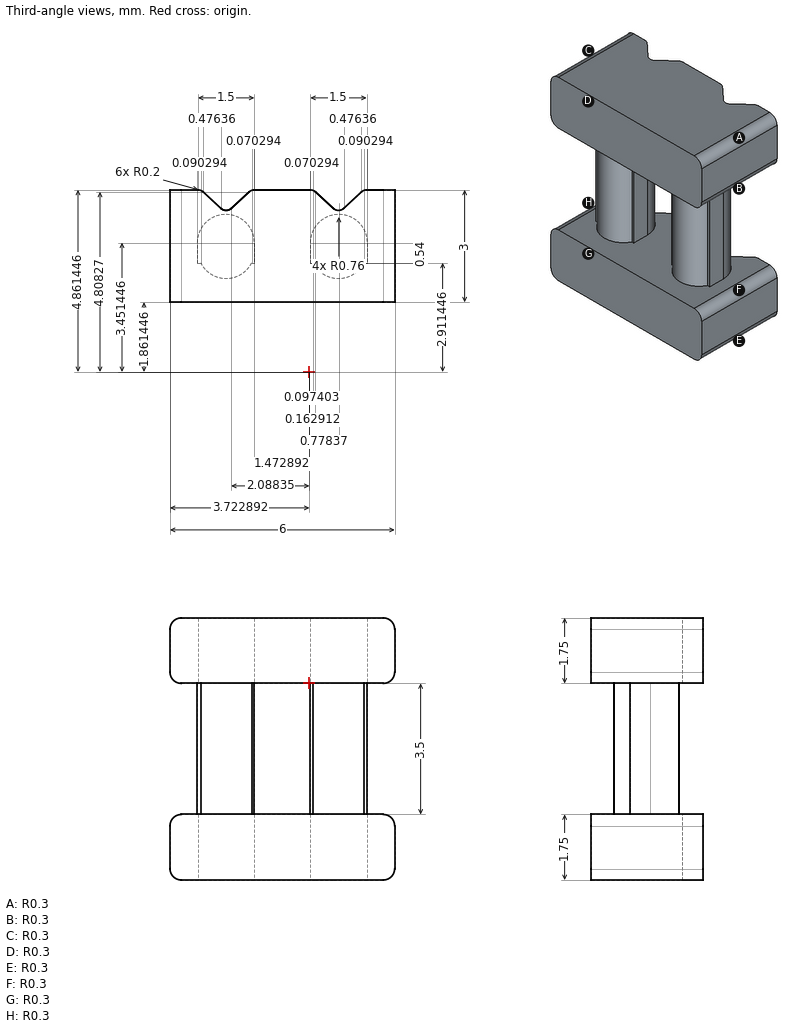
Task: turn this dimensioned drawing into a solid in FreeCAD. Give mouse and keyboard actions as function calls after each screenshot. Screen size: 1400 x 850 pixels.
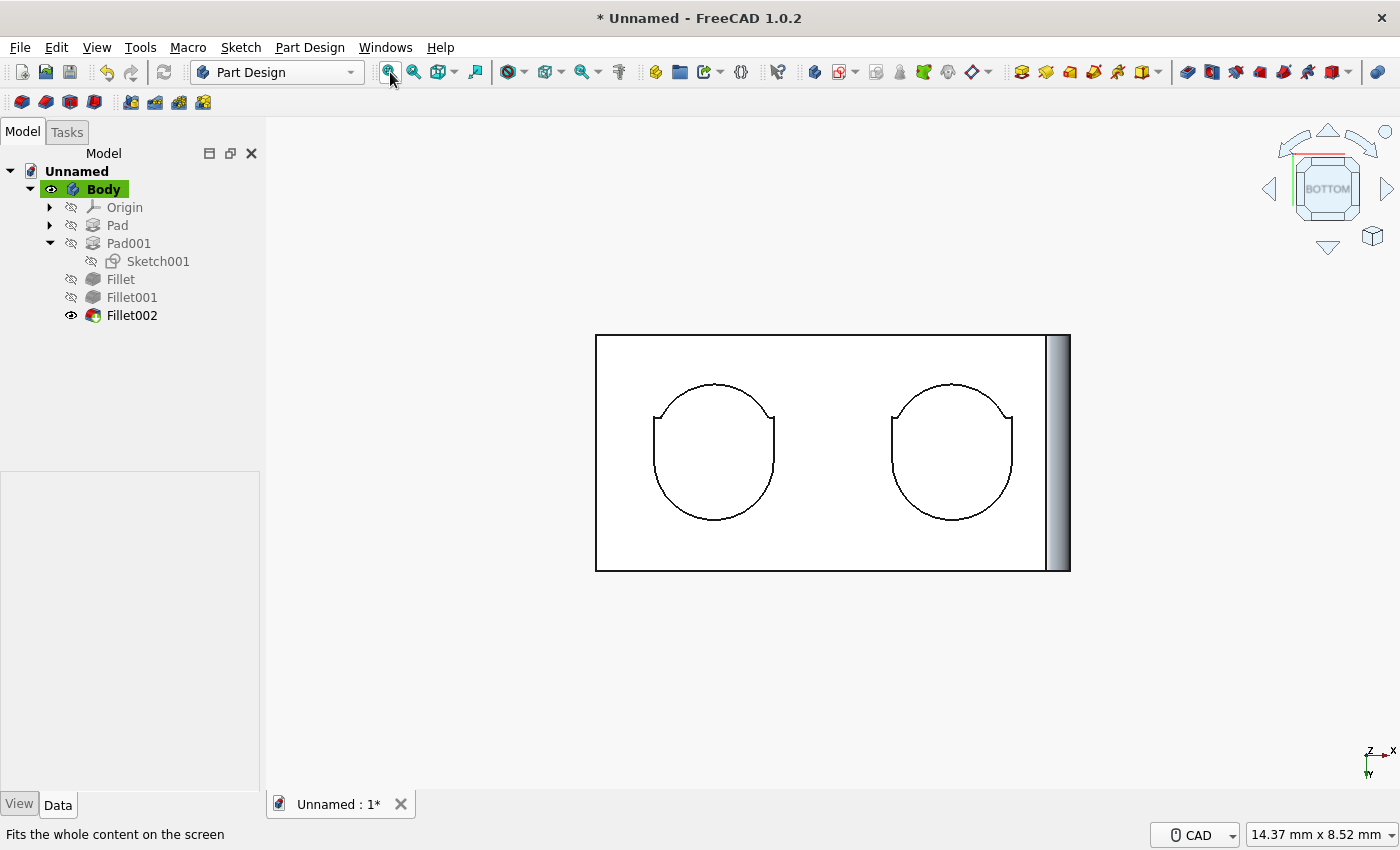
click(596, 452)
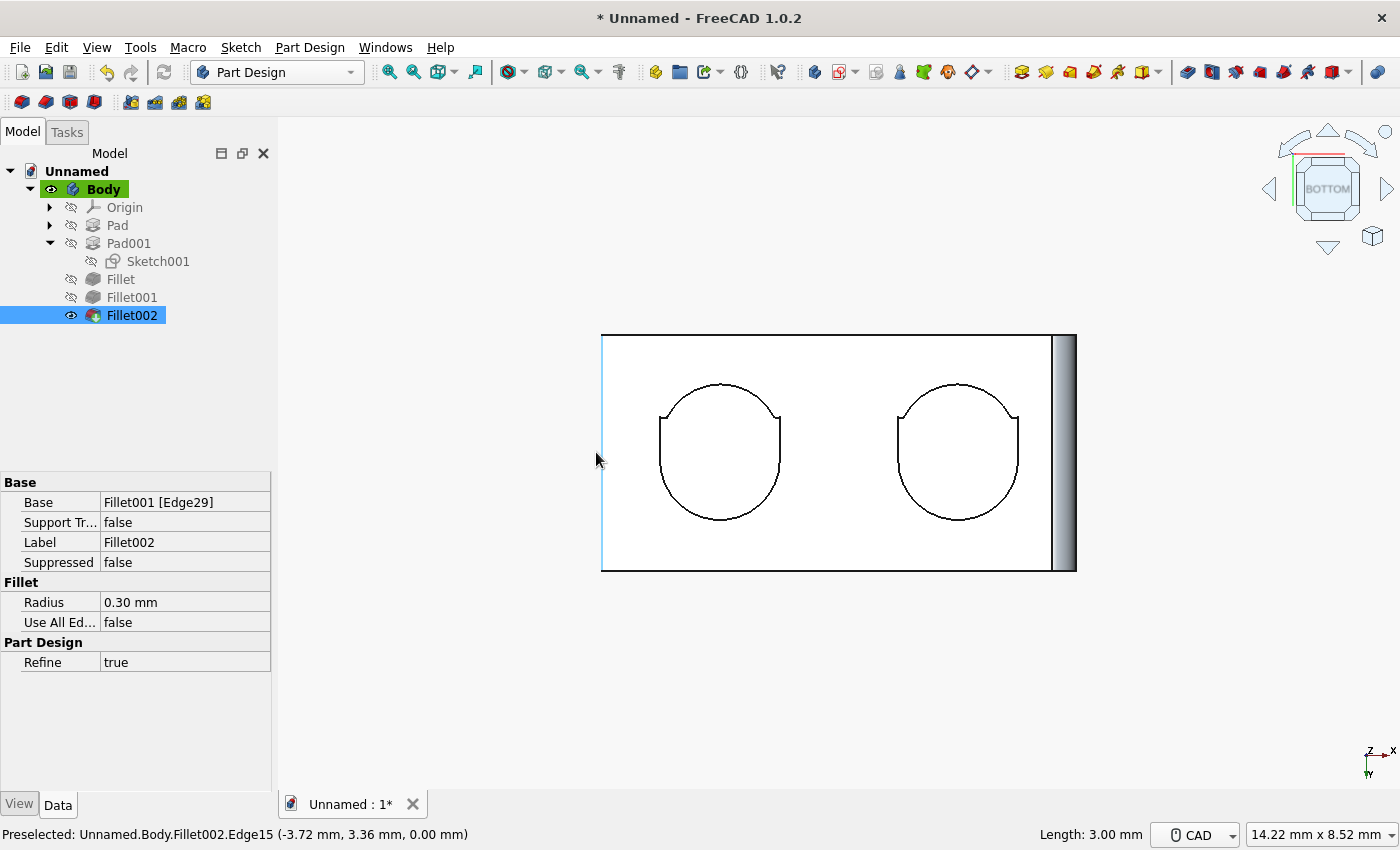
click(22, 102)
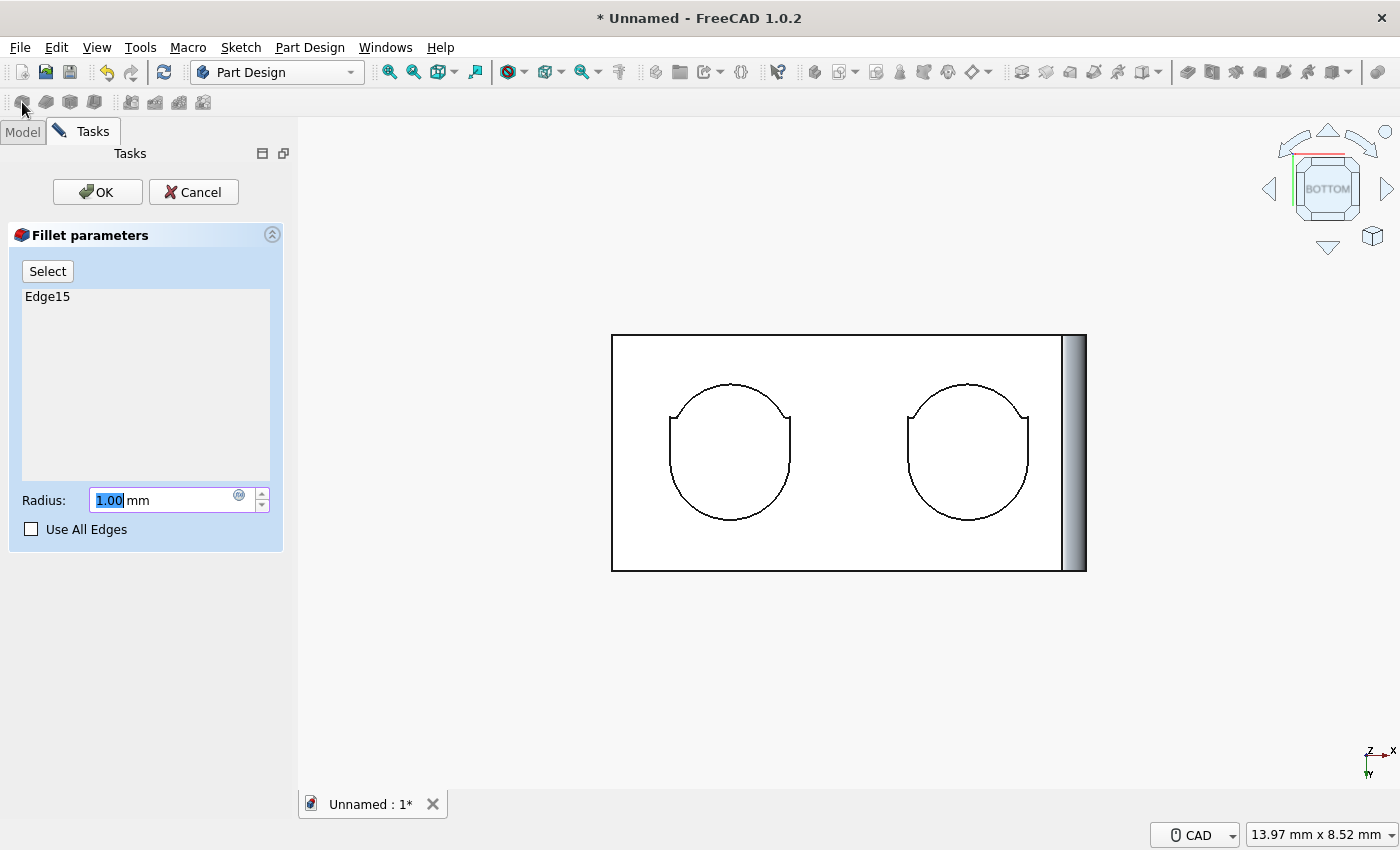
text(0.3)
key(Tab)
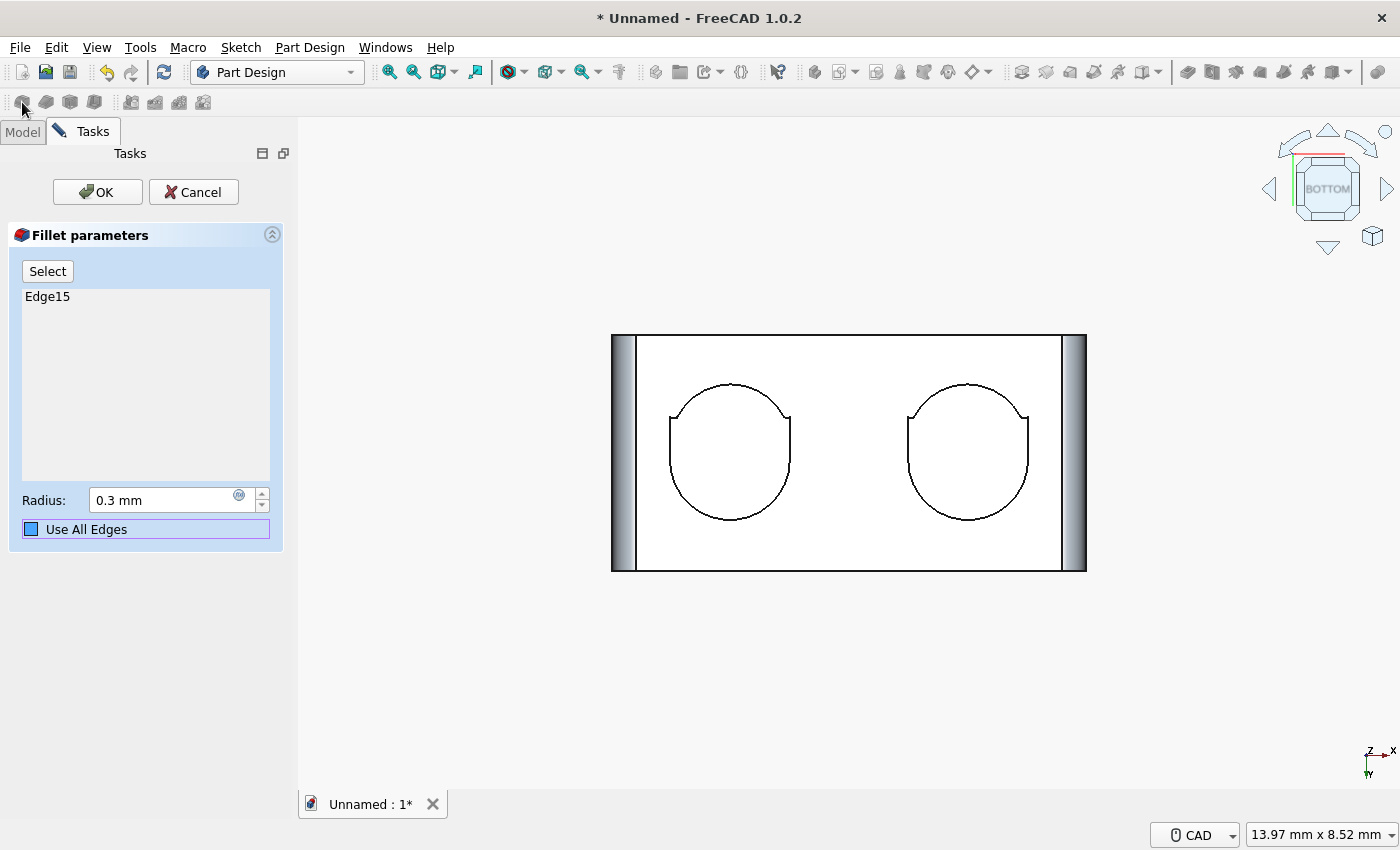
click(98, 192)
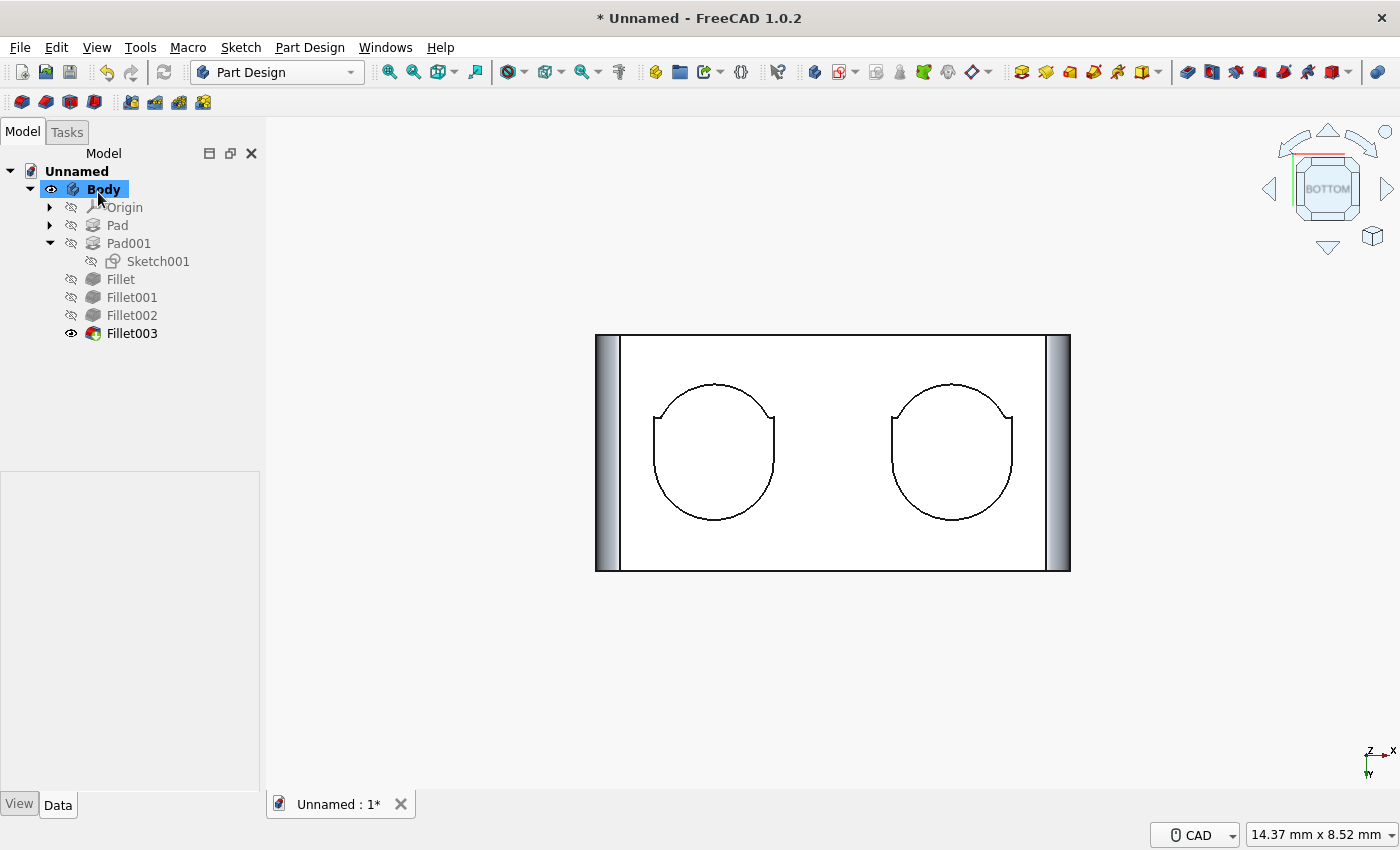
key(v)
key(f)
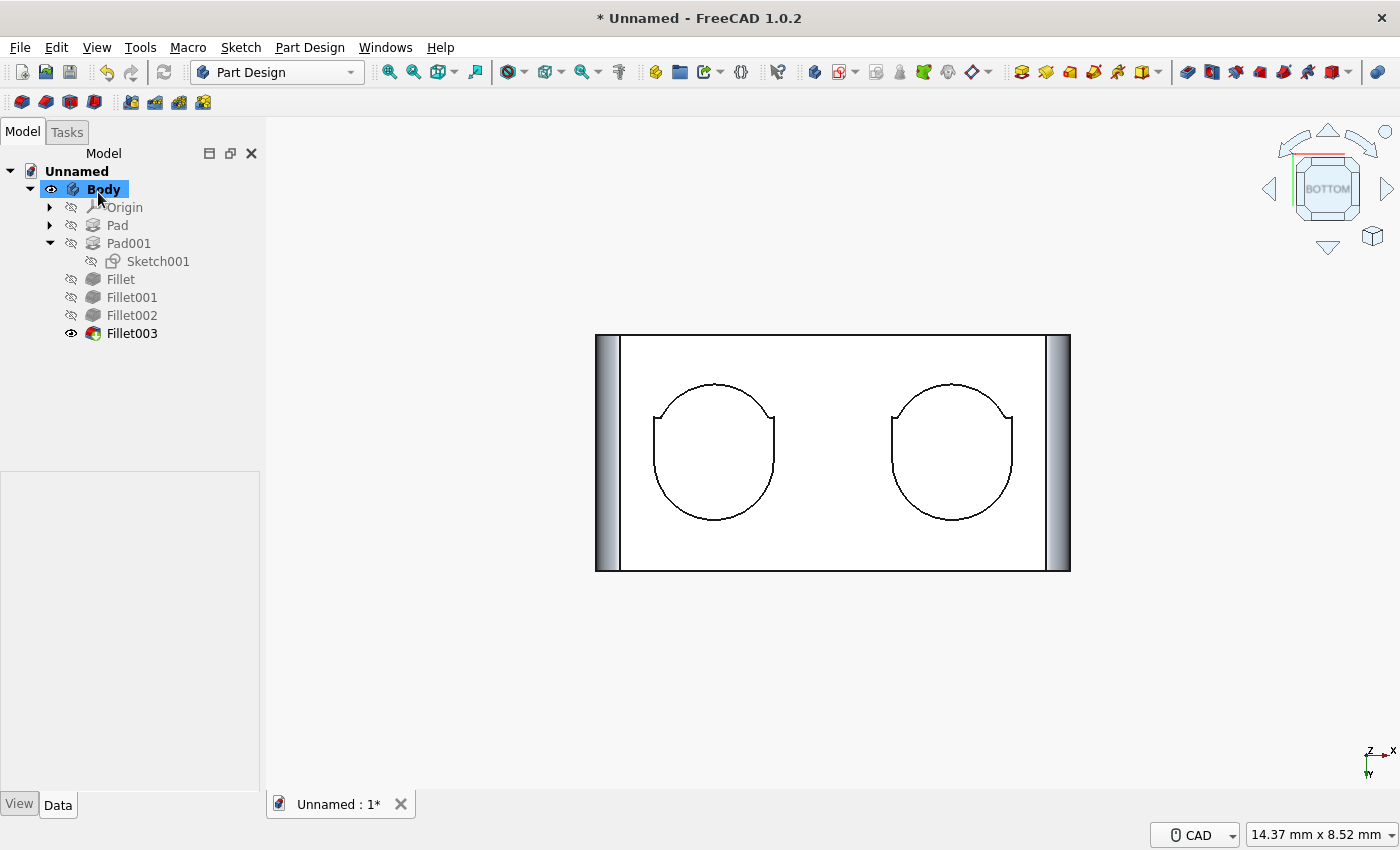
click(714, 451)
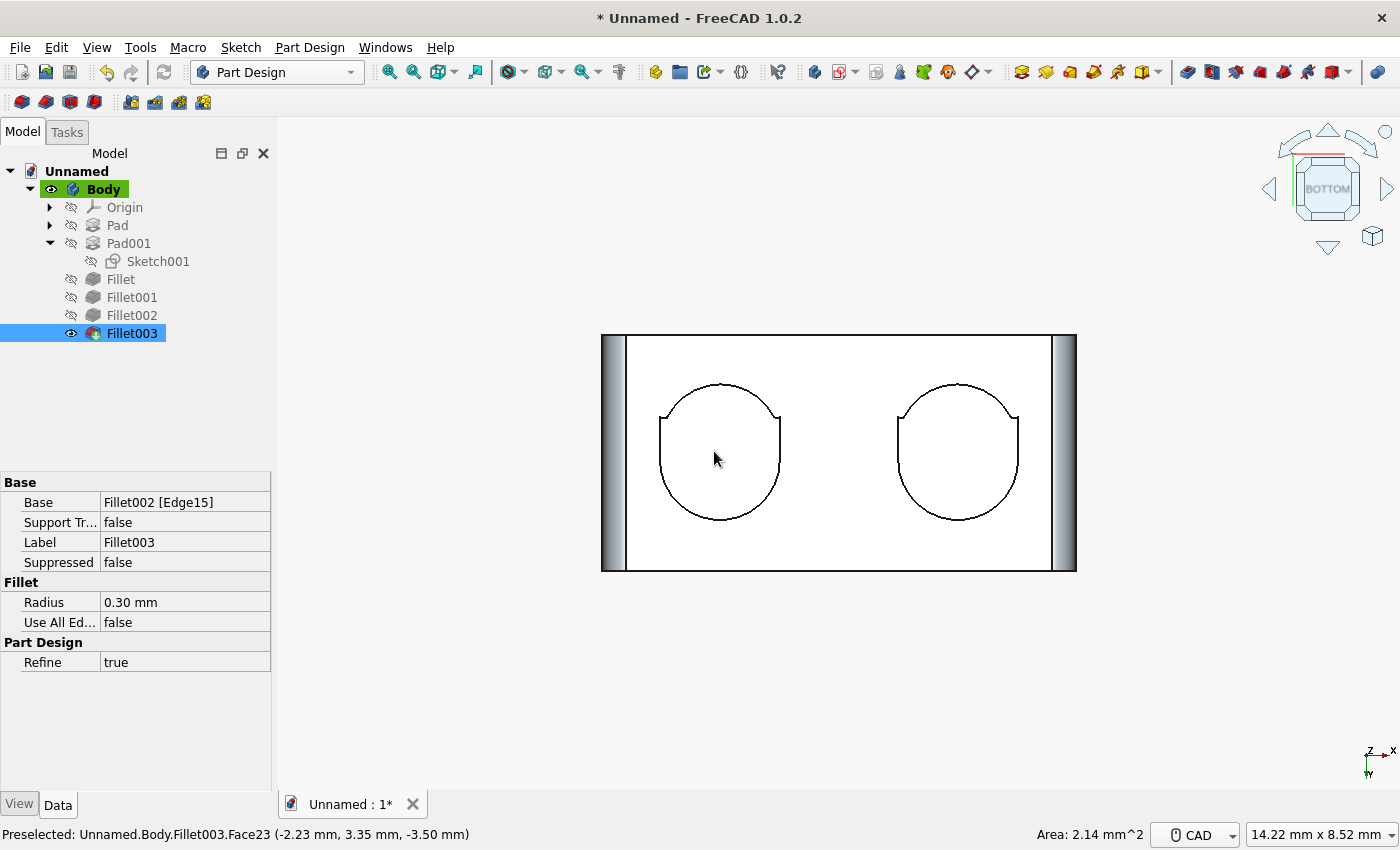
click(840, 72)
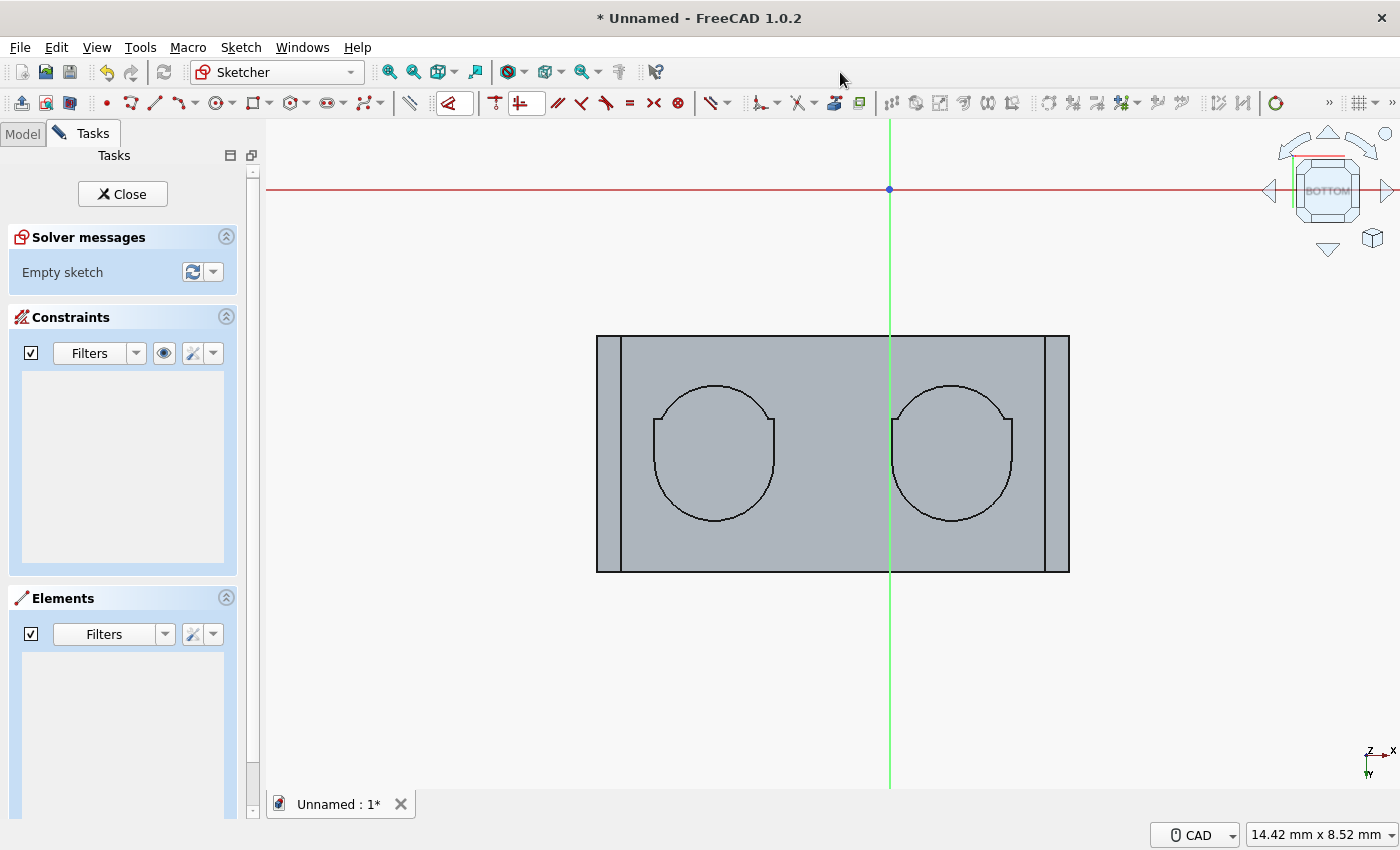
key(g)
key(r)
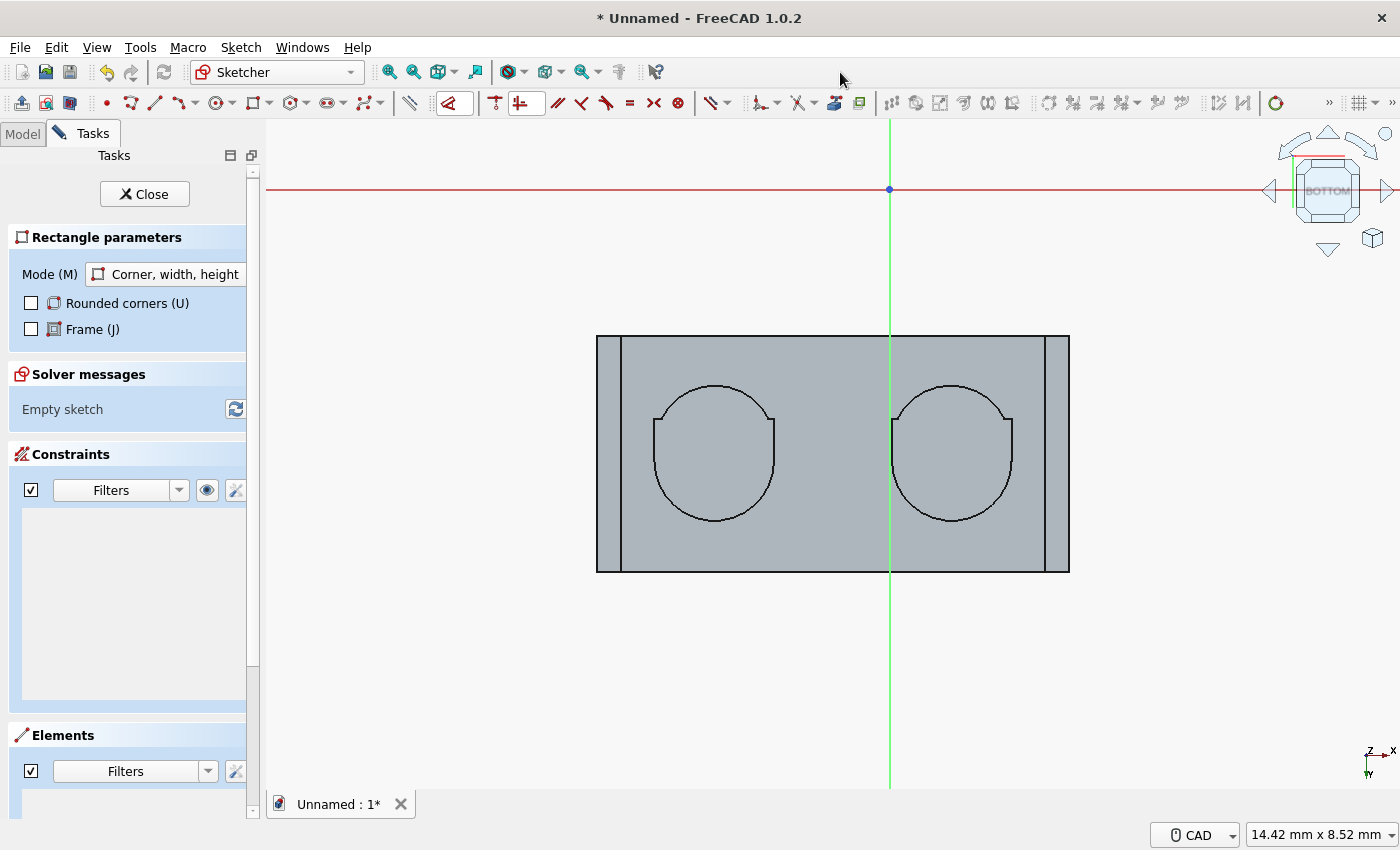
click(597, 336)
move(1069, 572)